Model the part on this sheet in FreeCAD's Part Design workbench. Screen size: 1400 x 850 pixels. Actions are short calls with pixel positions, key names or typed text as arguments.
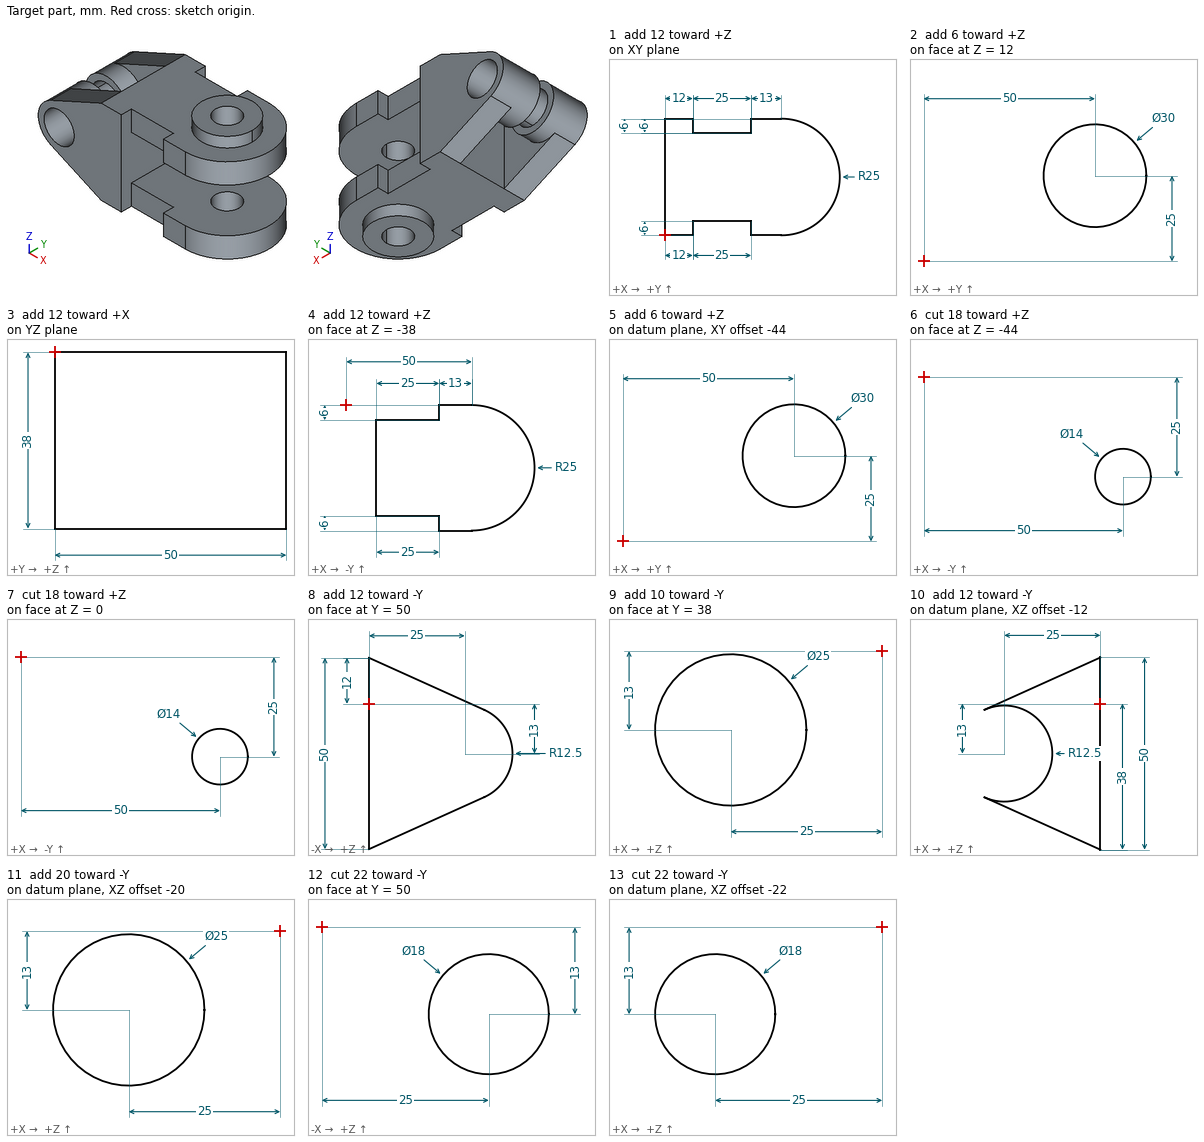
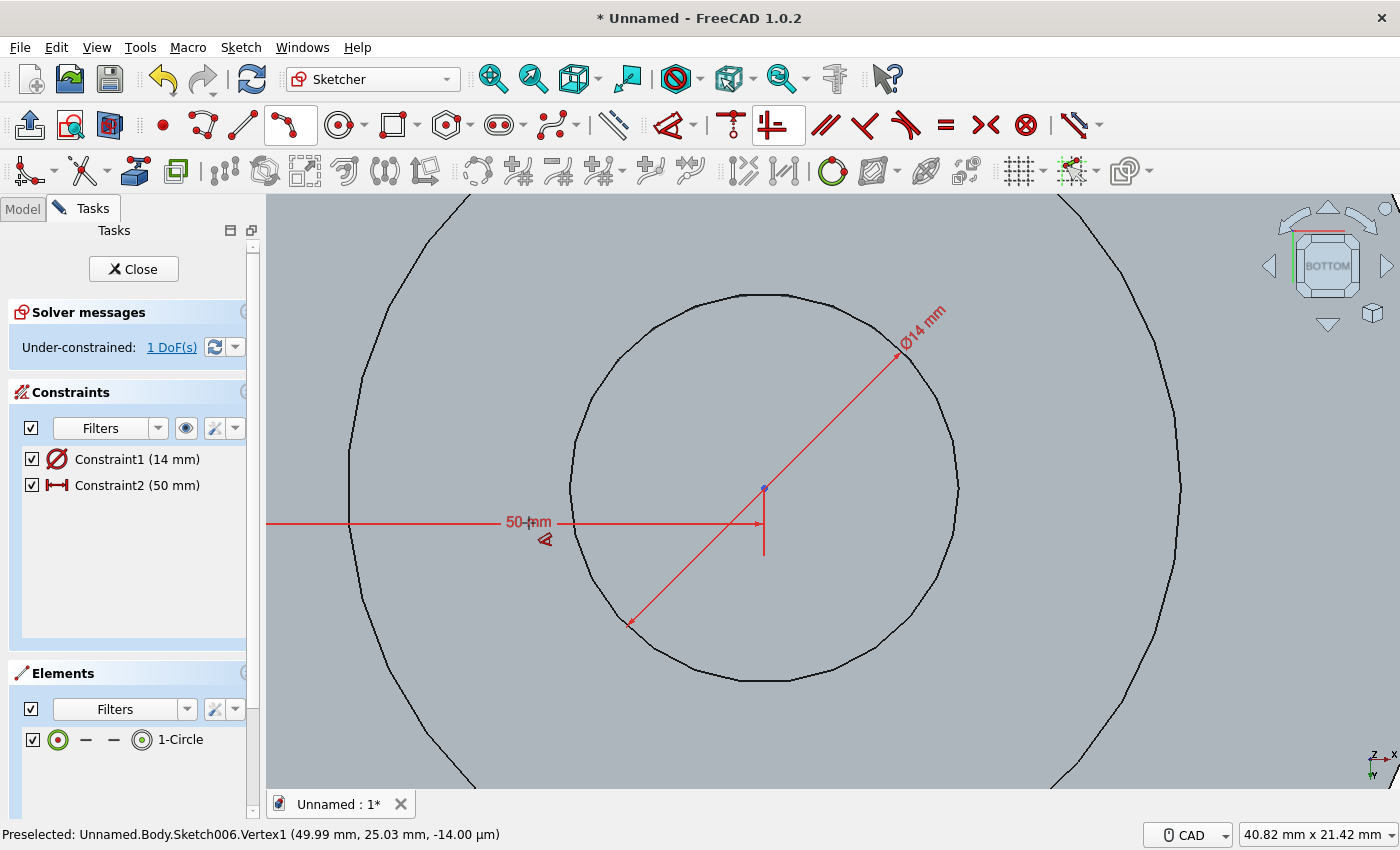
click(764, 489)
click(798, 355)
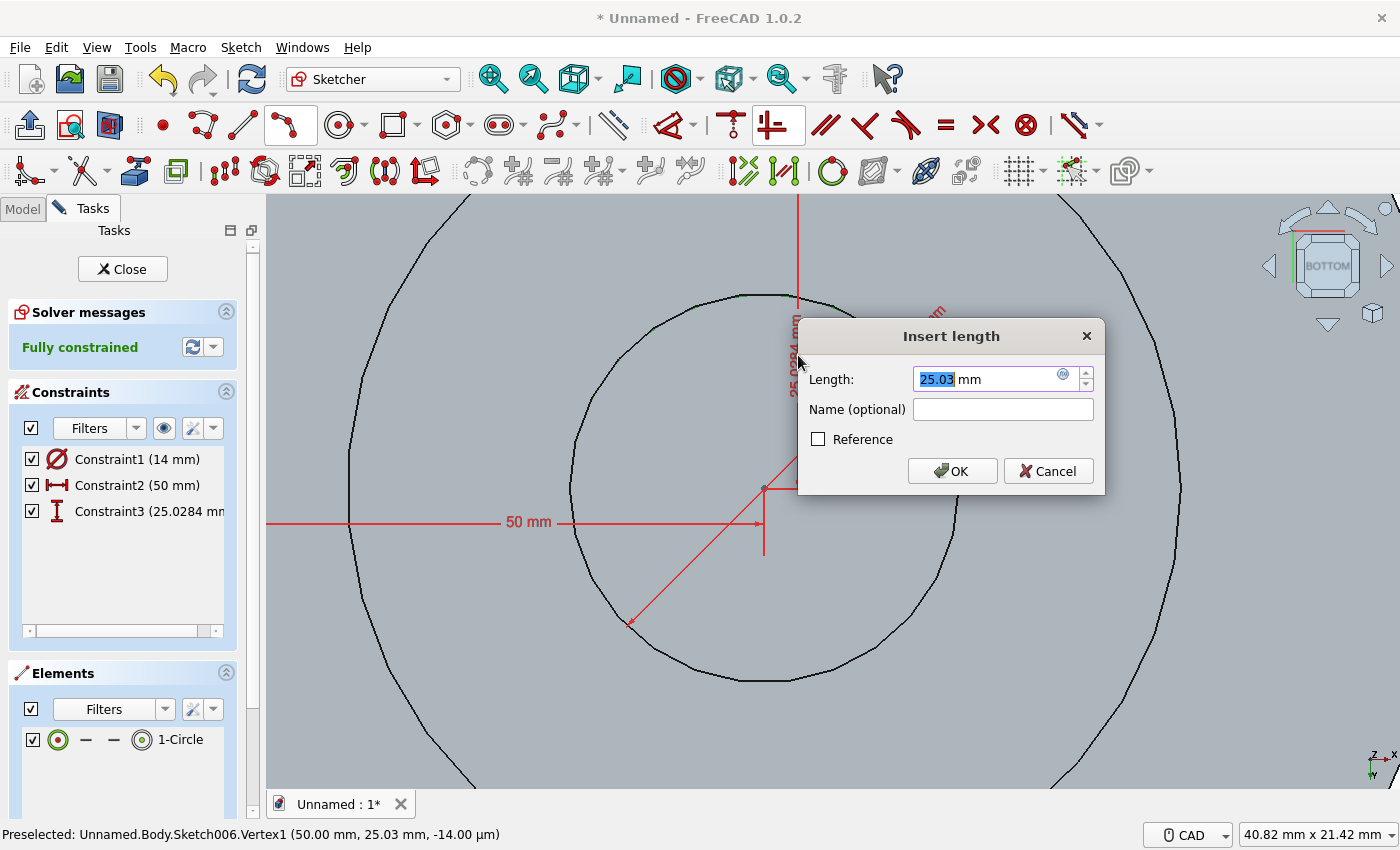
text(25)
key(Return)
key(Escape)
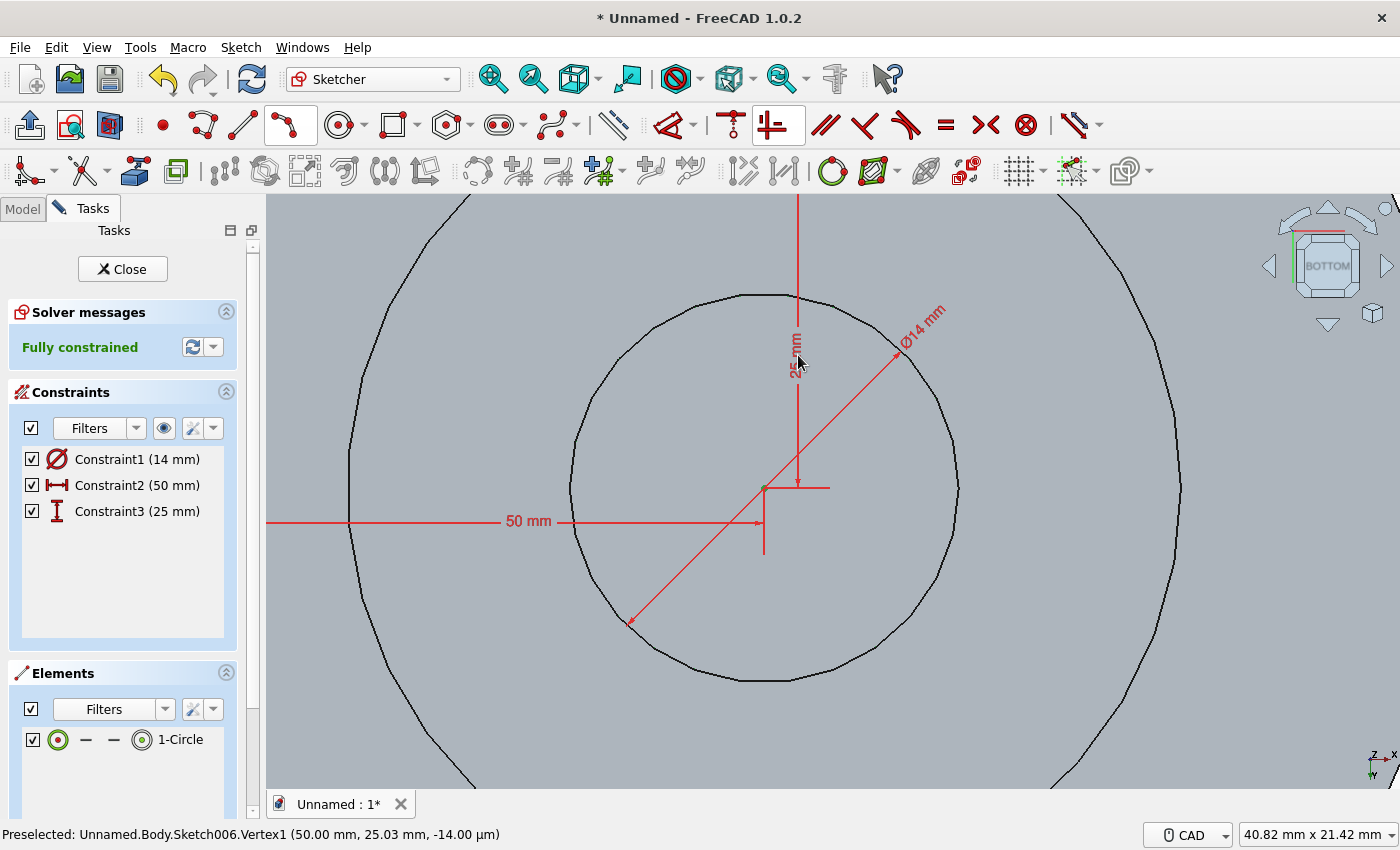
click(123, 269)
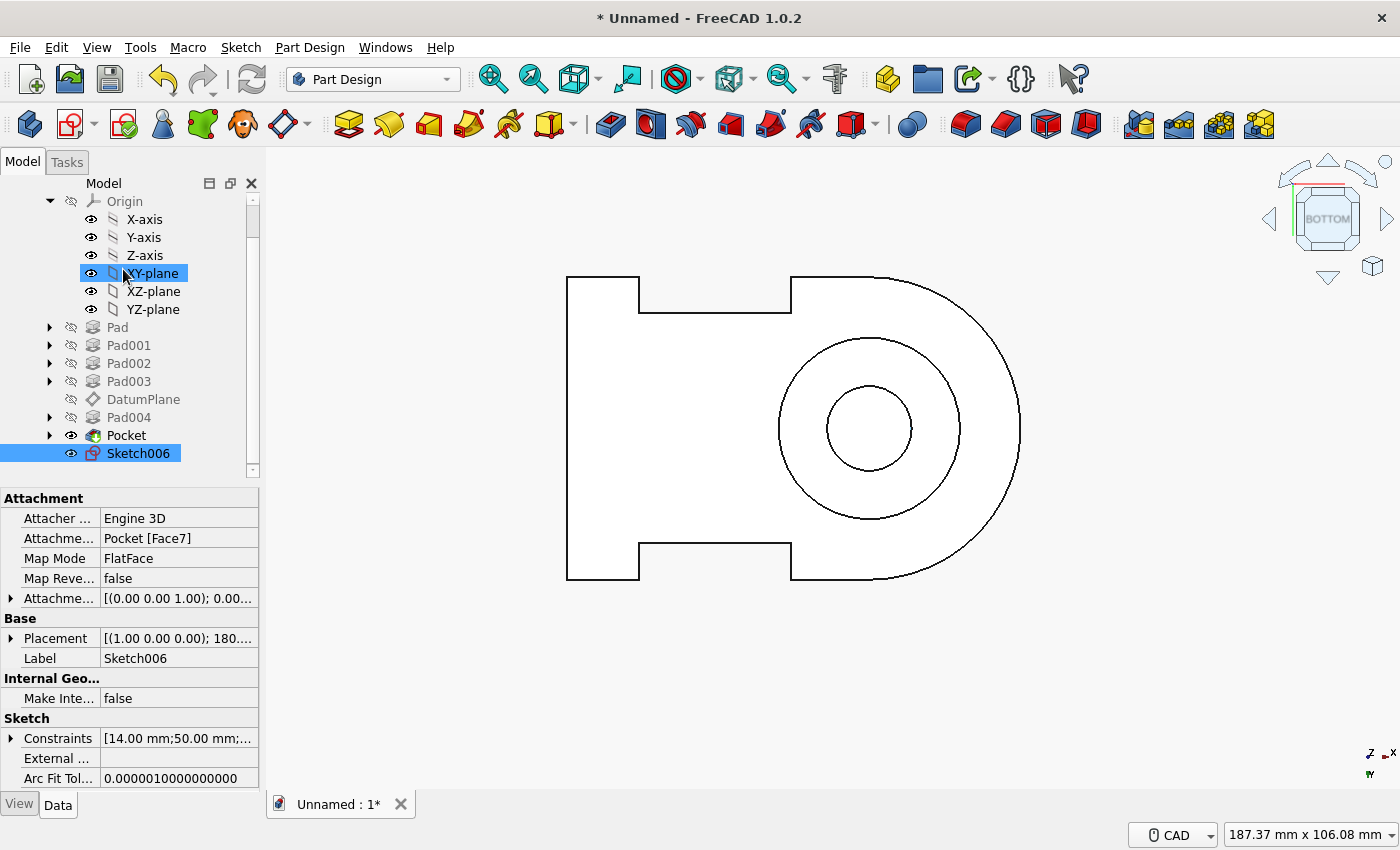
click(612, 124)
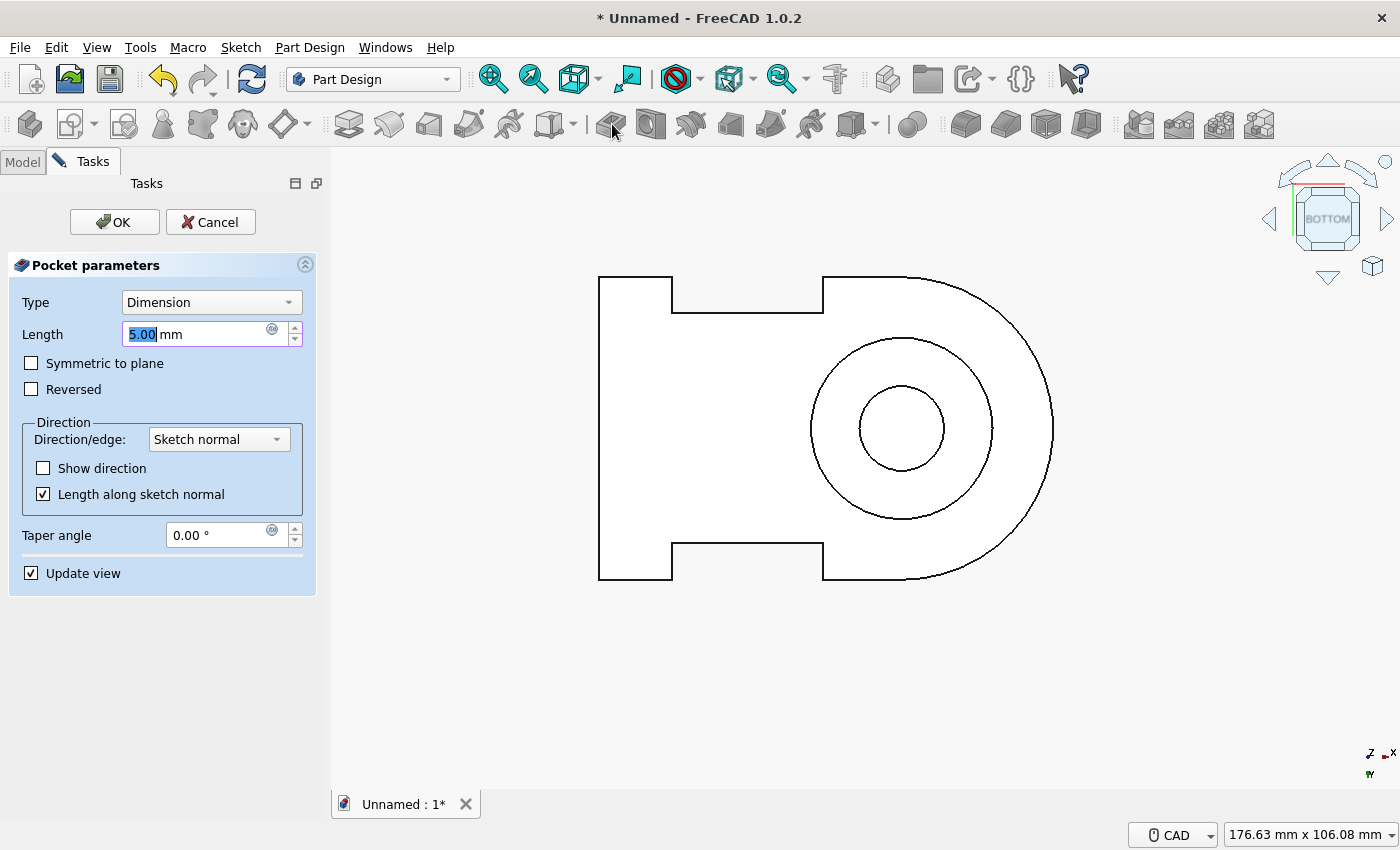
text(18)
key(Tab)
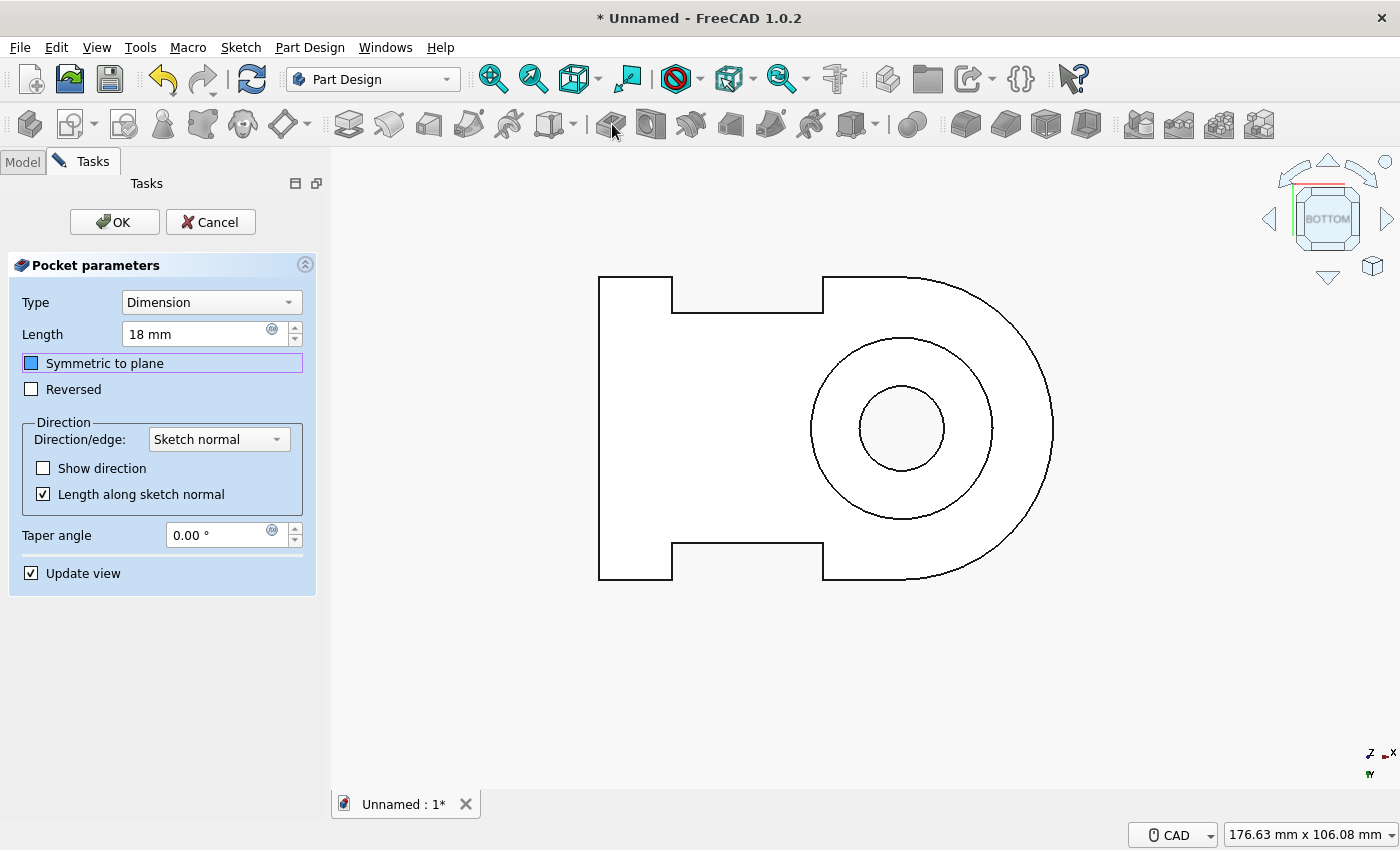
click(115, 222)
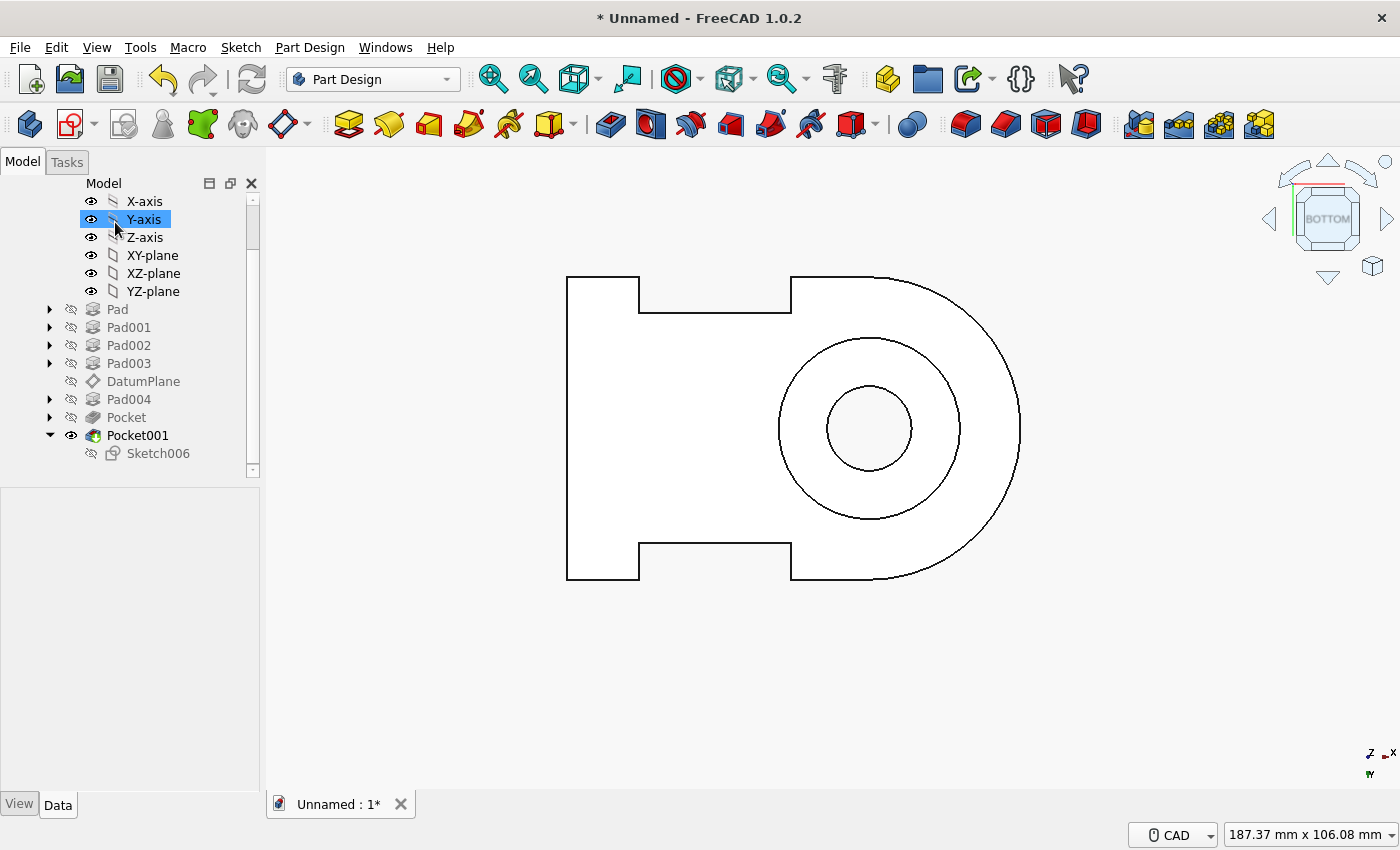
key(4)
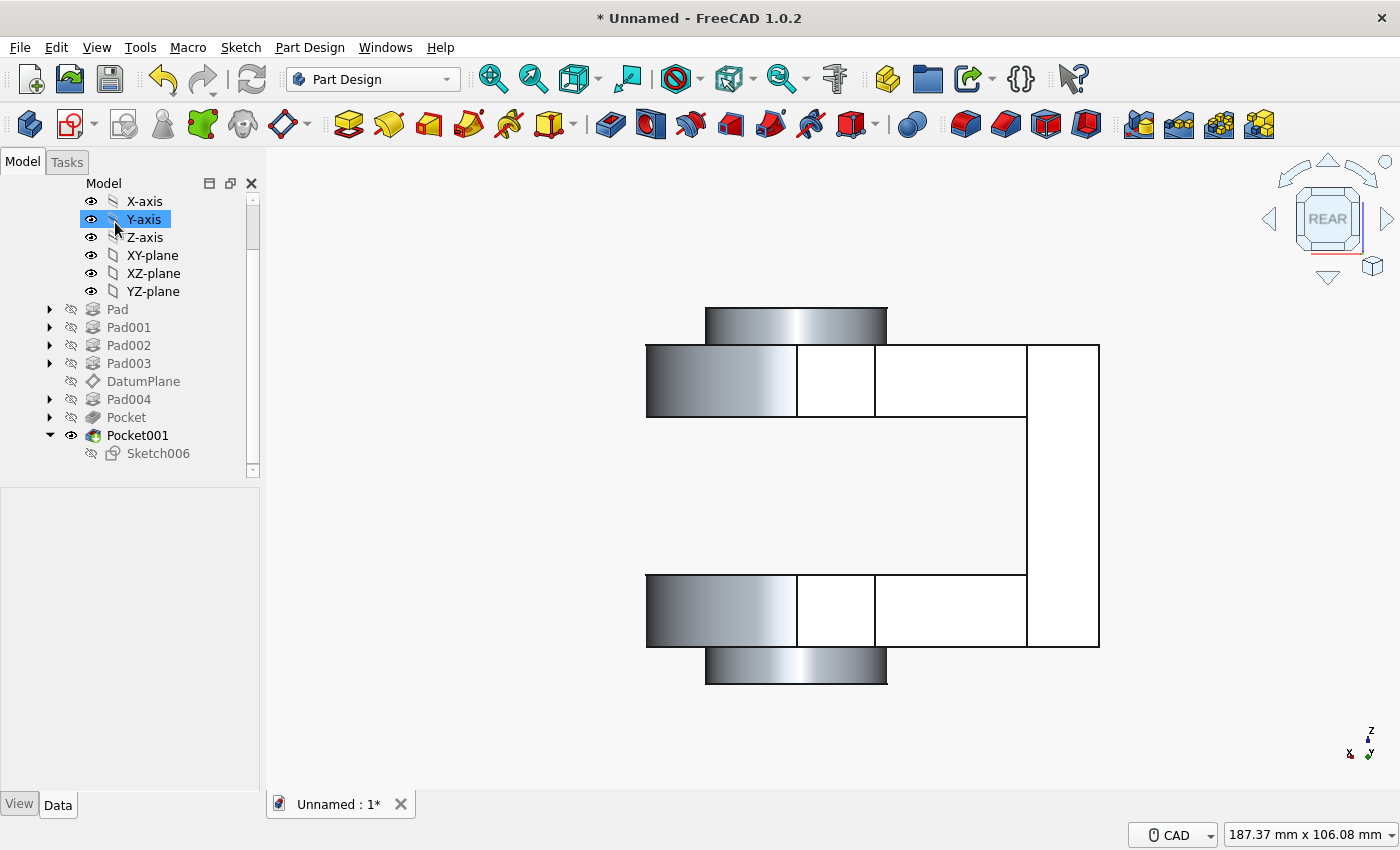
click(1063, 408)